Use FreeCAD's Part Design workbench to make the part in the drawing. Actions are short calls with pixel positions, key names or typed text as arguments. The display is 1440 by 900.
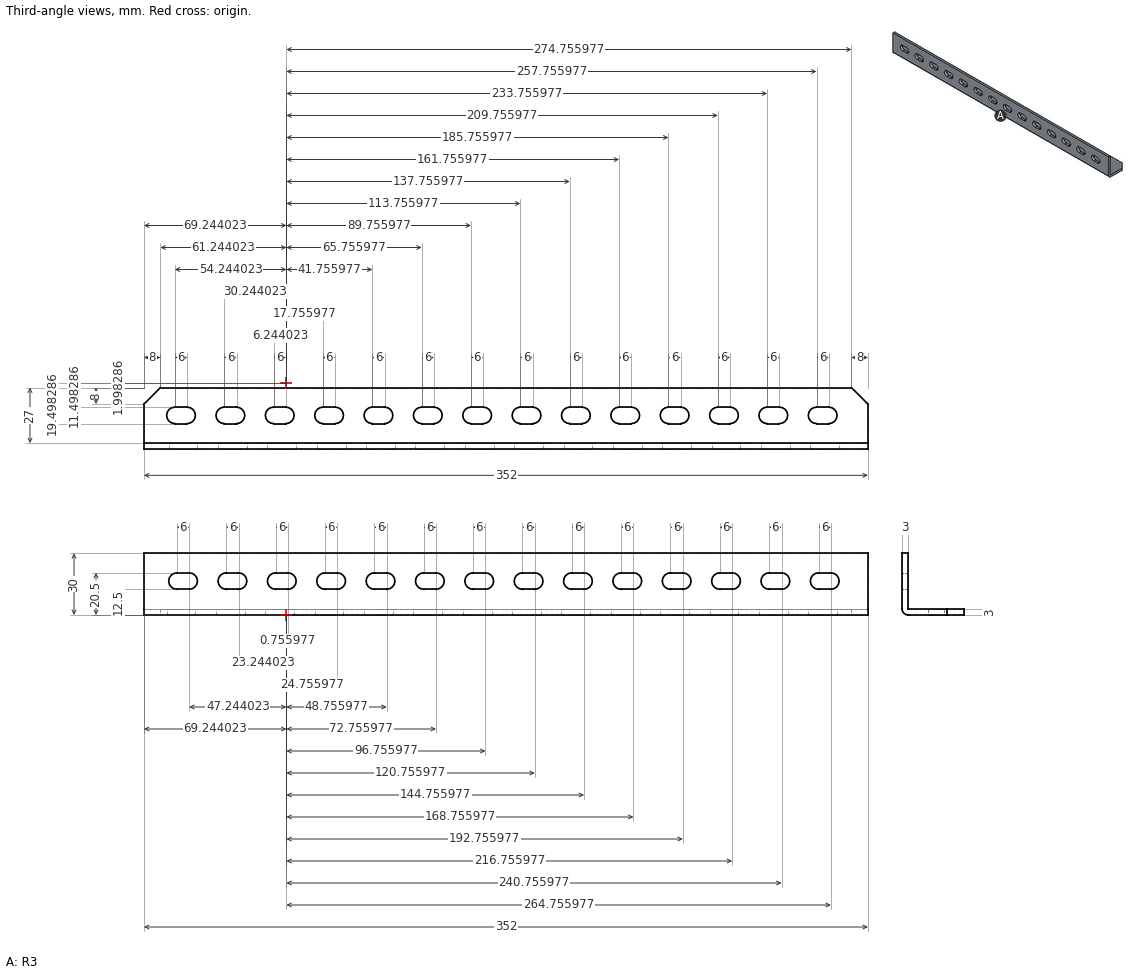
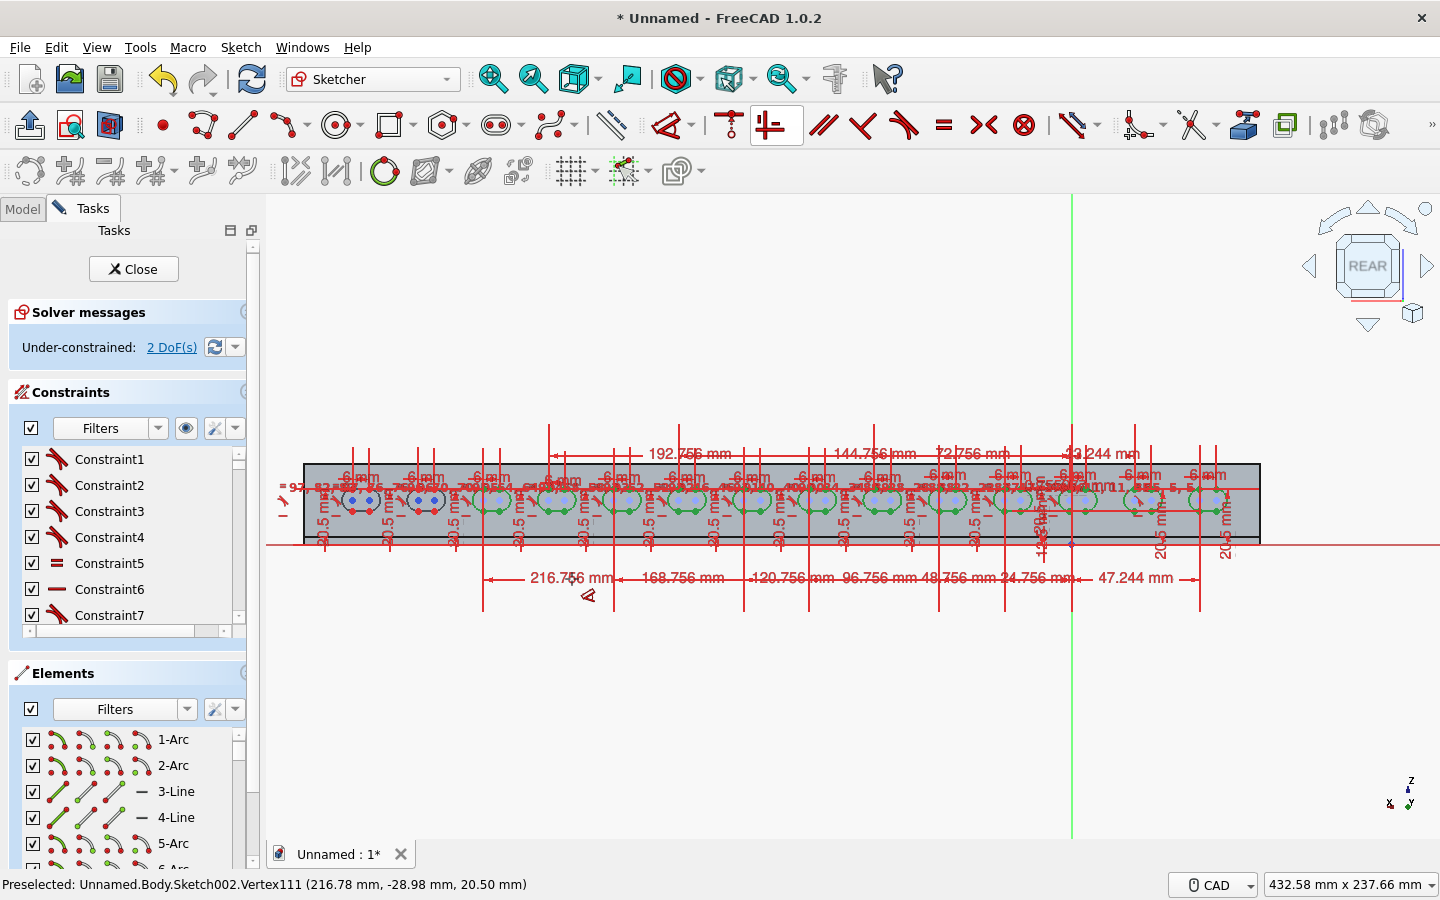
click(418, 489)
click(595, 455)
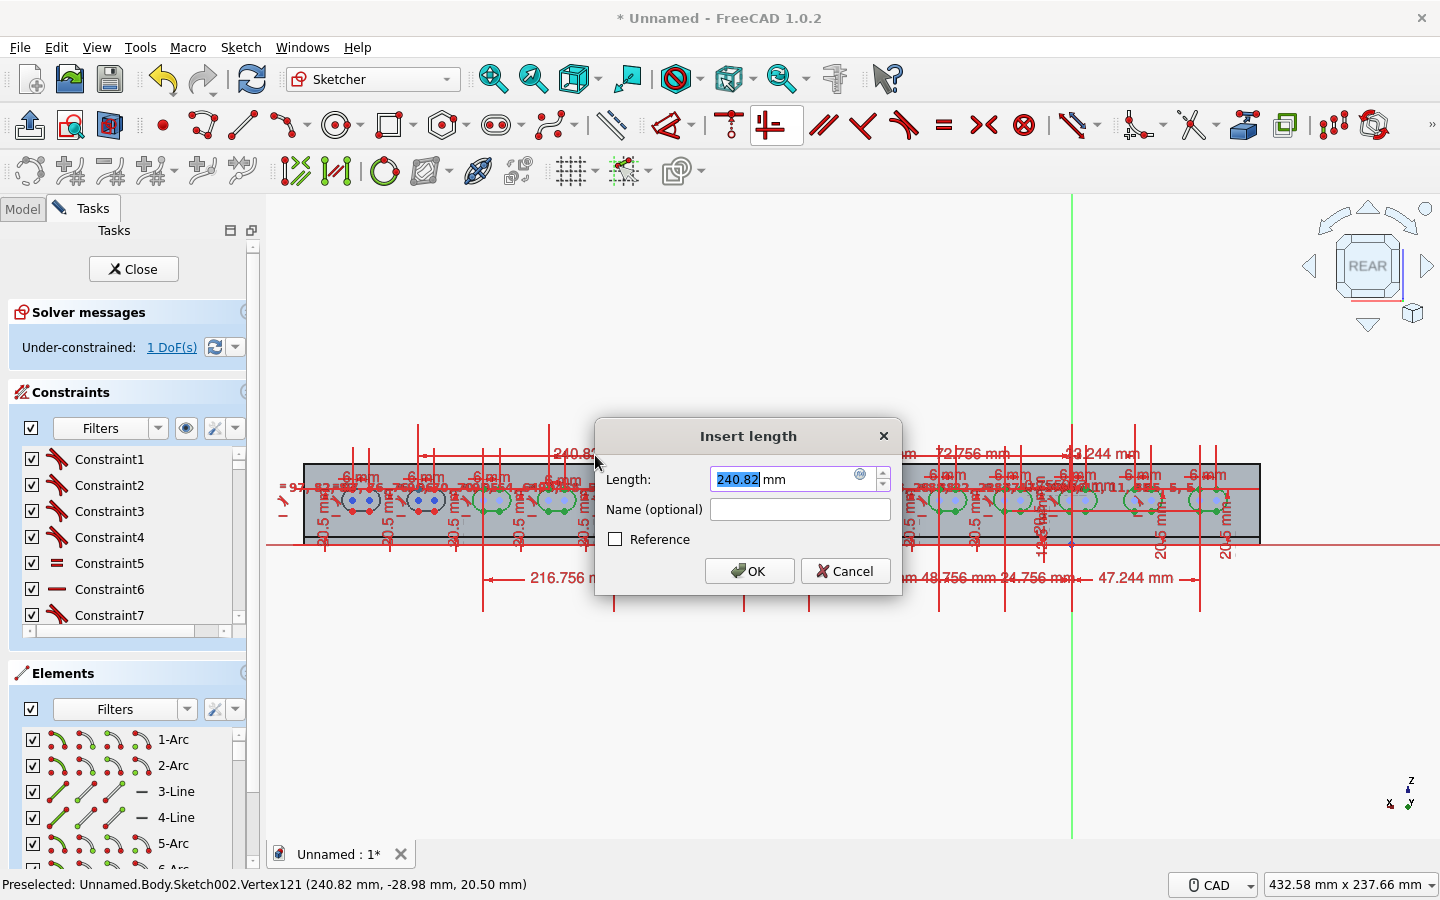
text(240.755977)
key(Return)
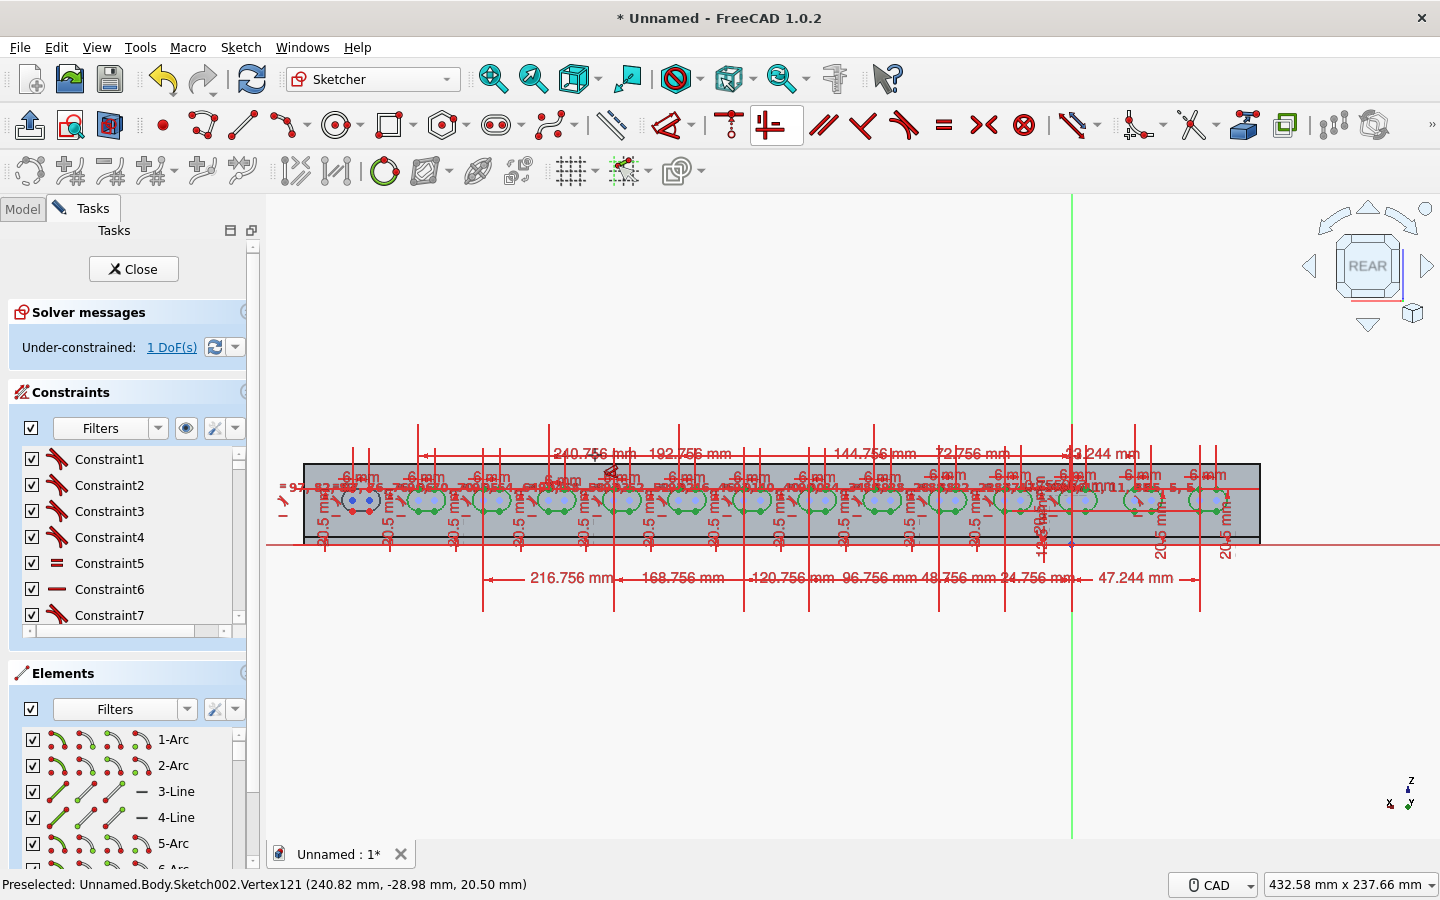
click(353, 489)
click(461, 579)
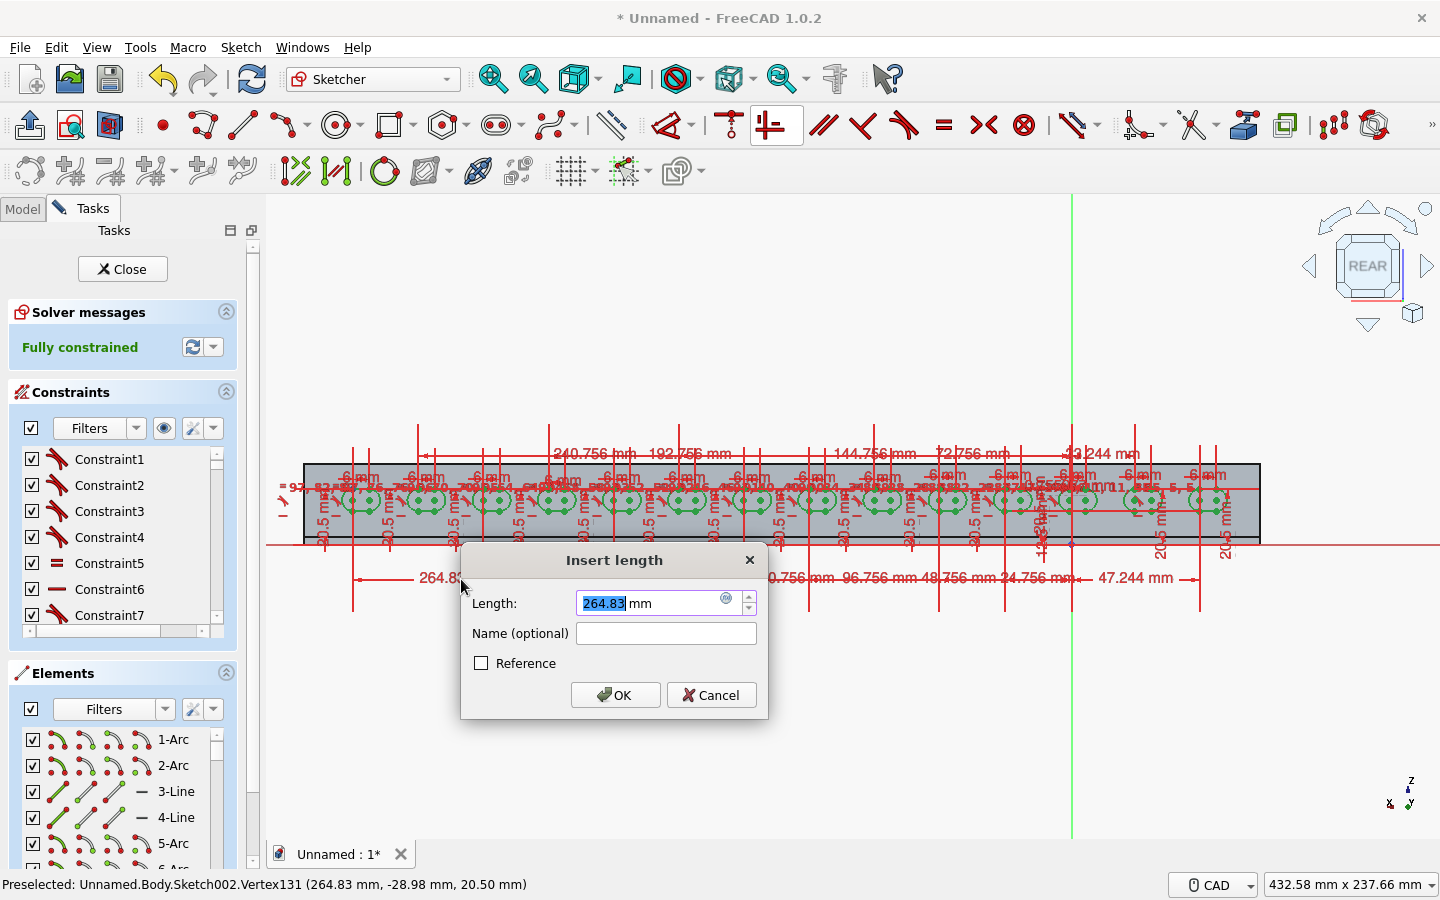
text(264.755977)
key(Return)
key(Escape)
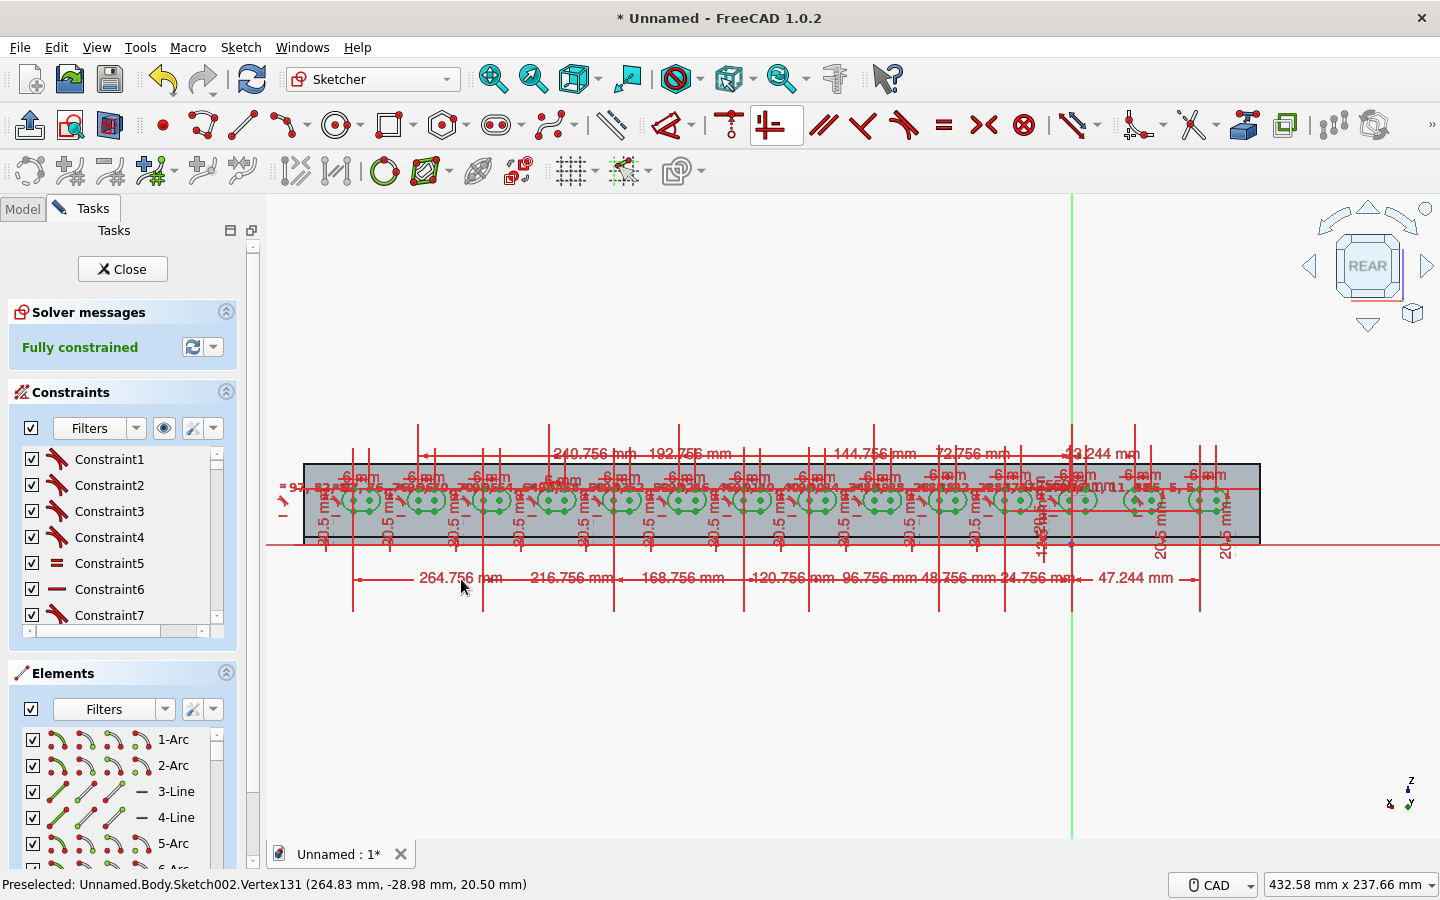
click(123, 269)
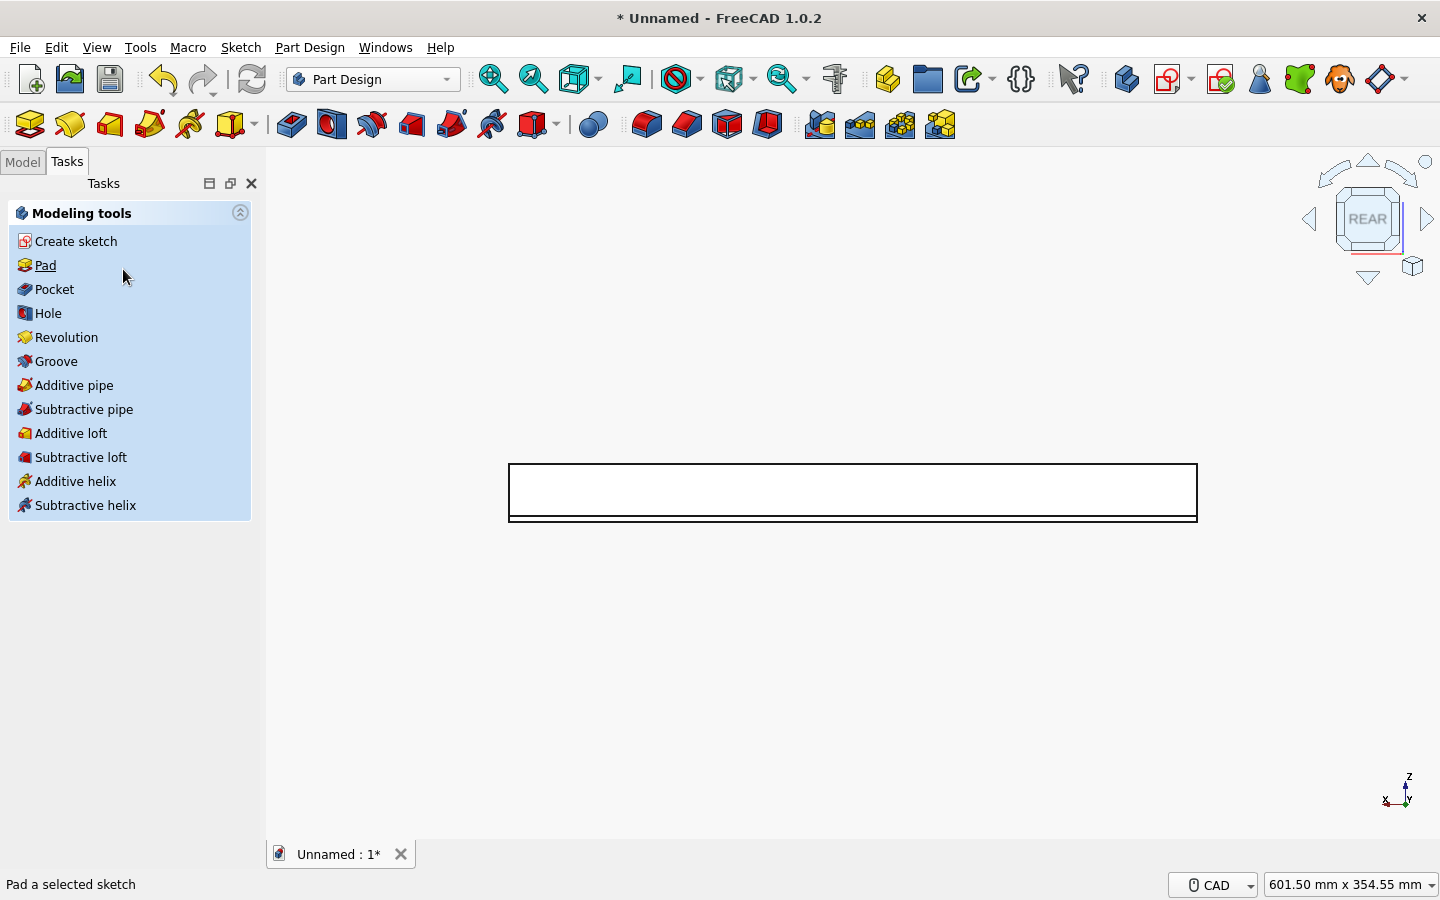
click(292, 124)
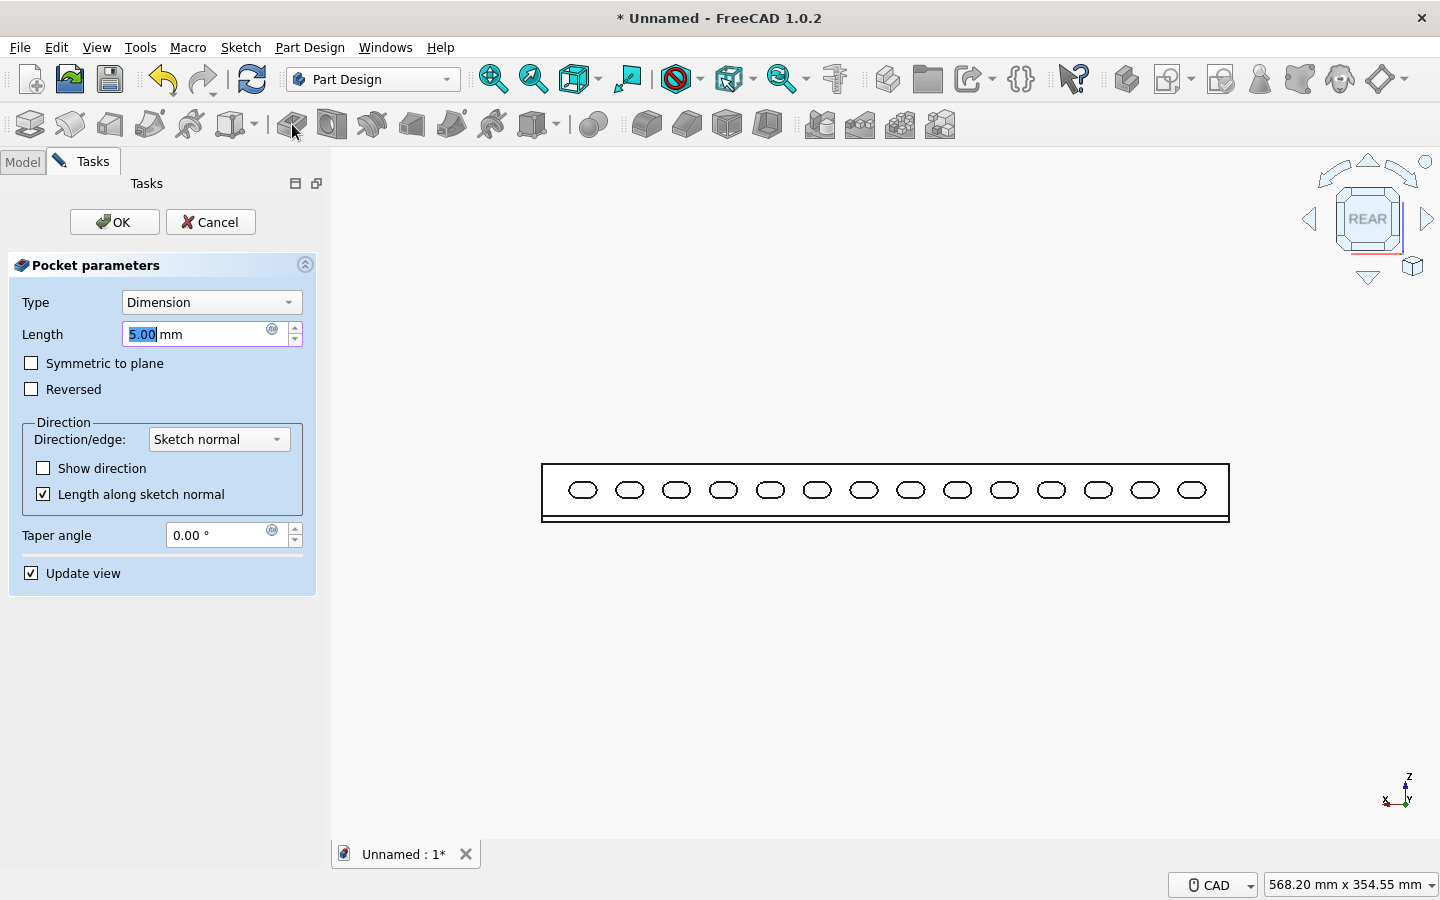
text(3)
key(Tab)